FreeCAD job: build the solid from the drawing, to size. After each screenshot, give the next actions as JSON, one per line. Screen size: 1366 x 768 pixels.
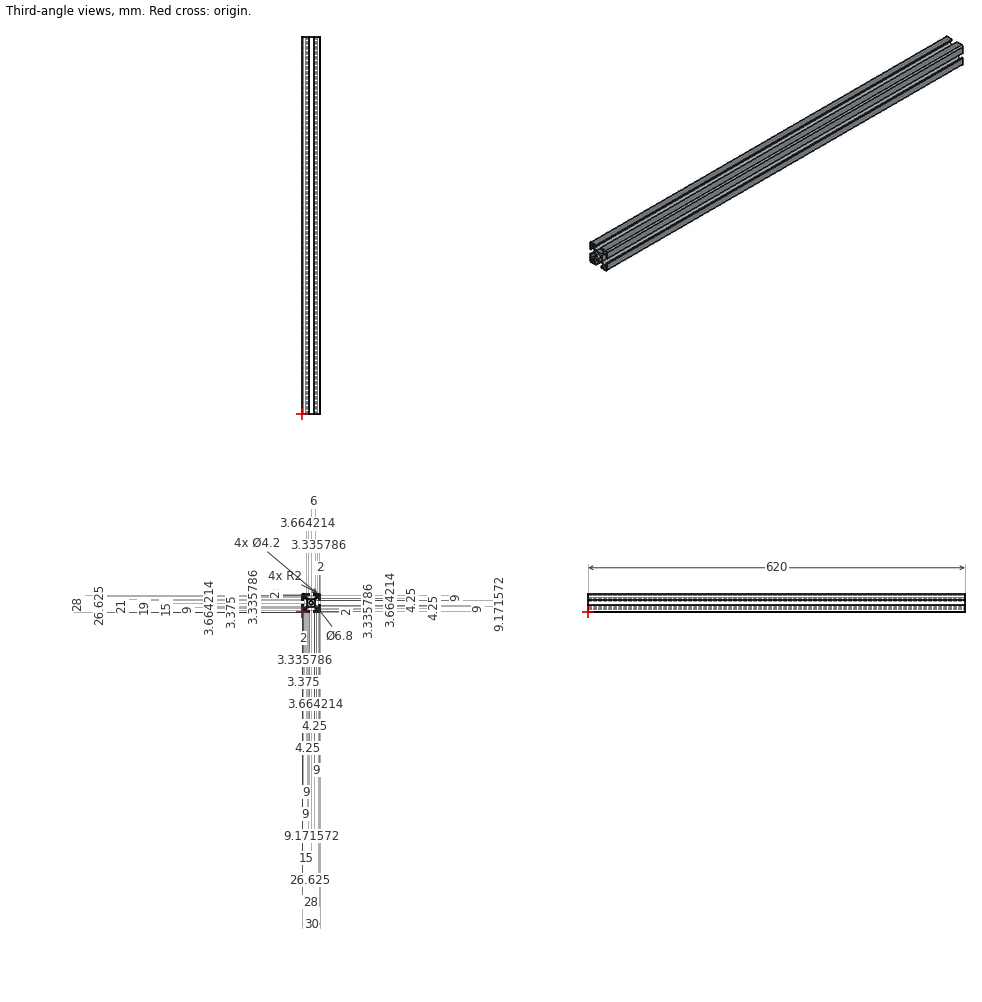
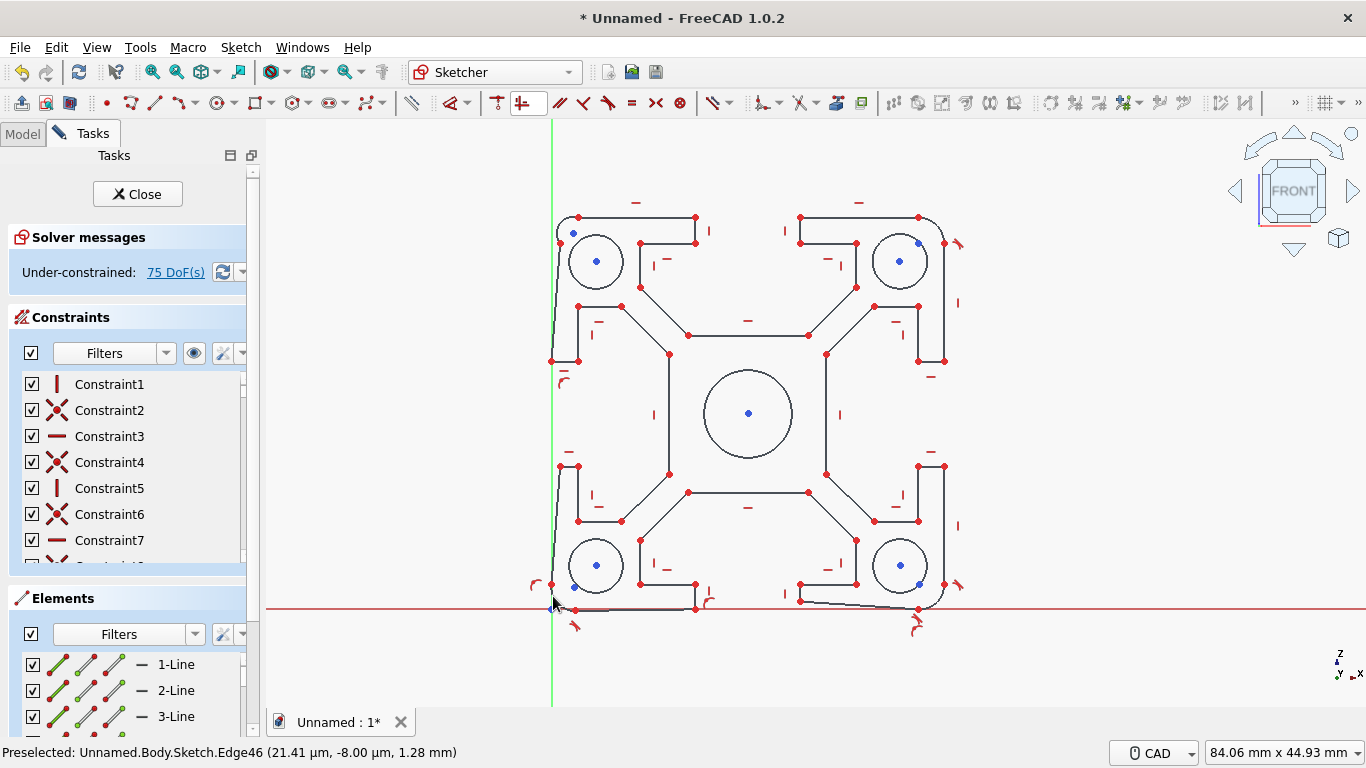
{"action": "left_click", "coordinate": [554, 549]}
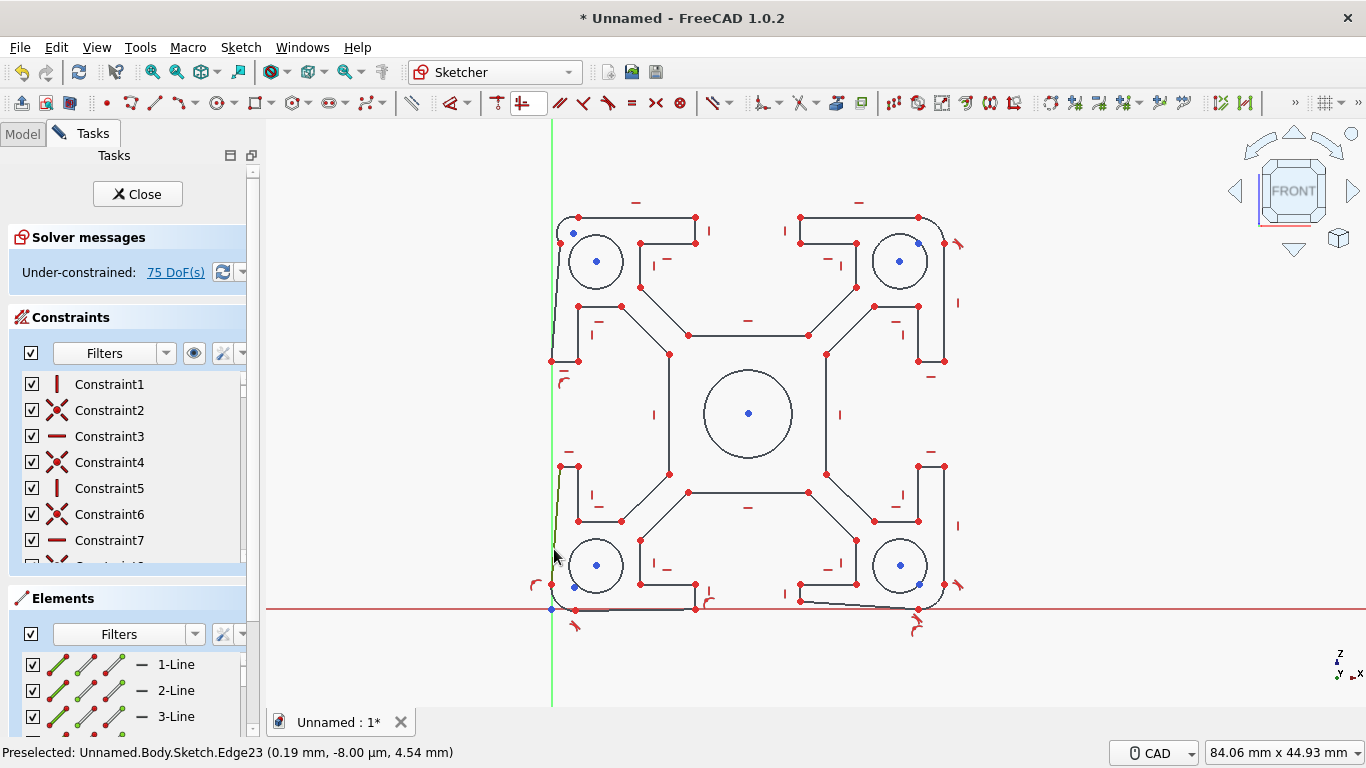
{"action": "left_click", "coordinate": [553, 596]}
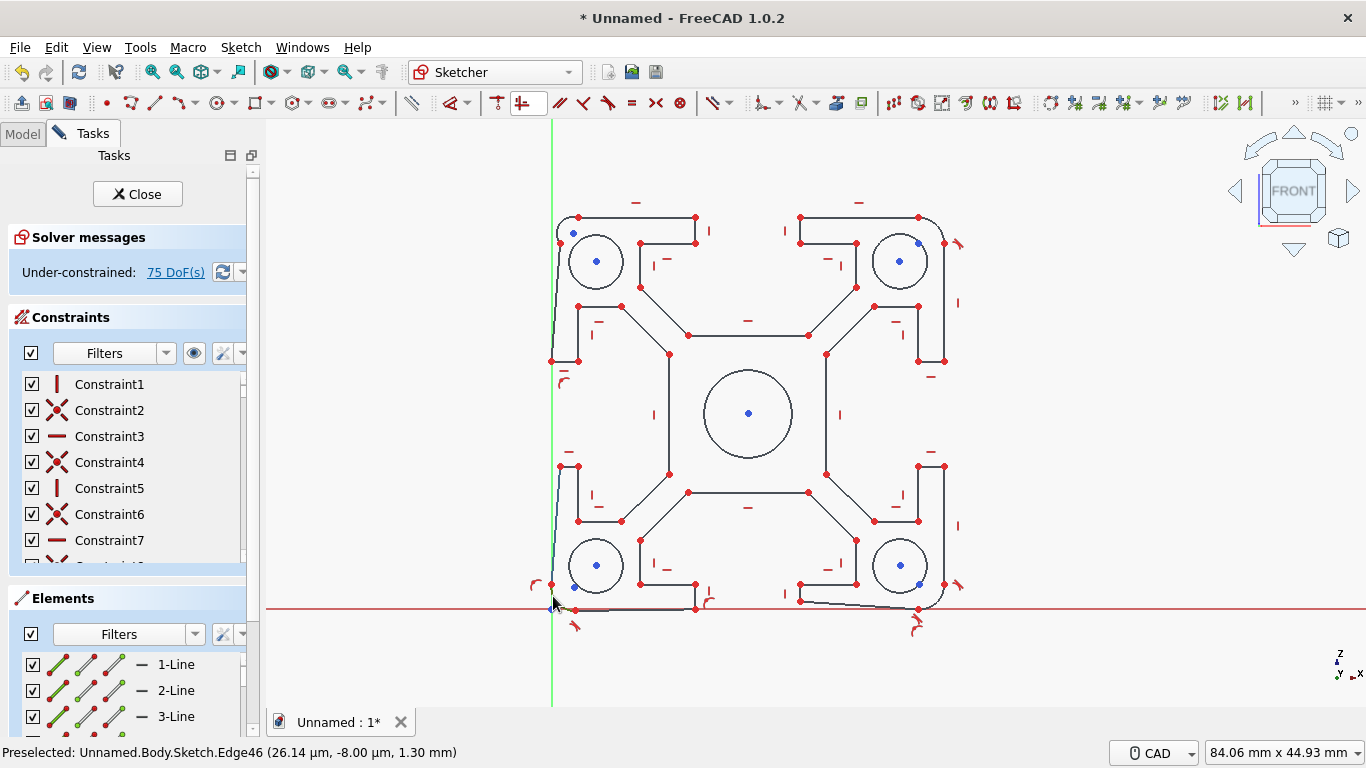
{"action": "key", "text": "t"}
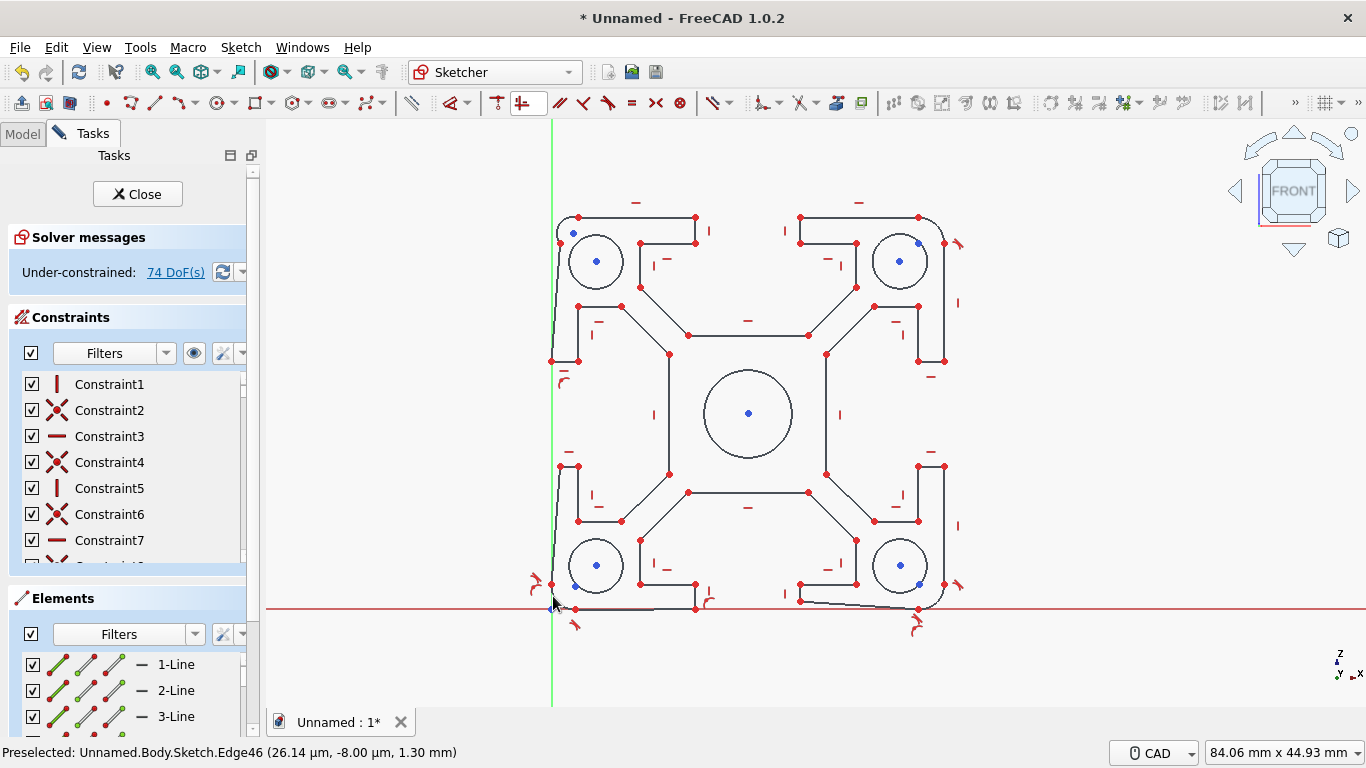
{"action": "left_click", "coordinate": [554, 326]}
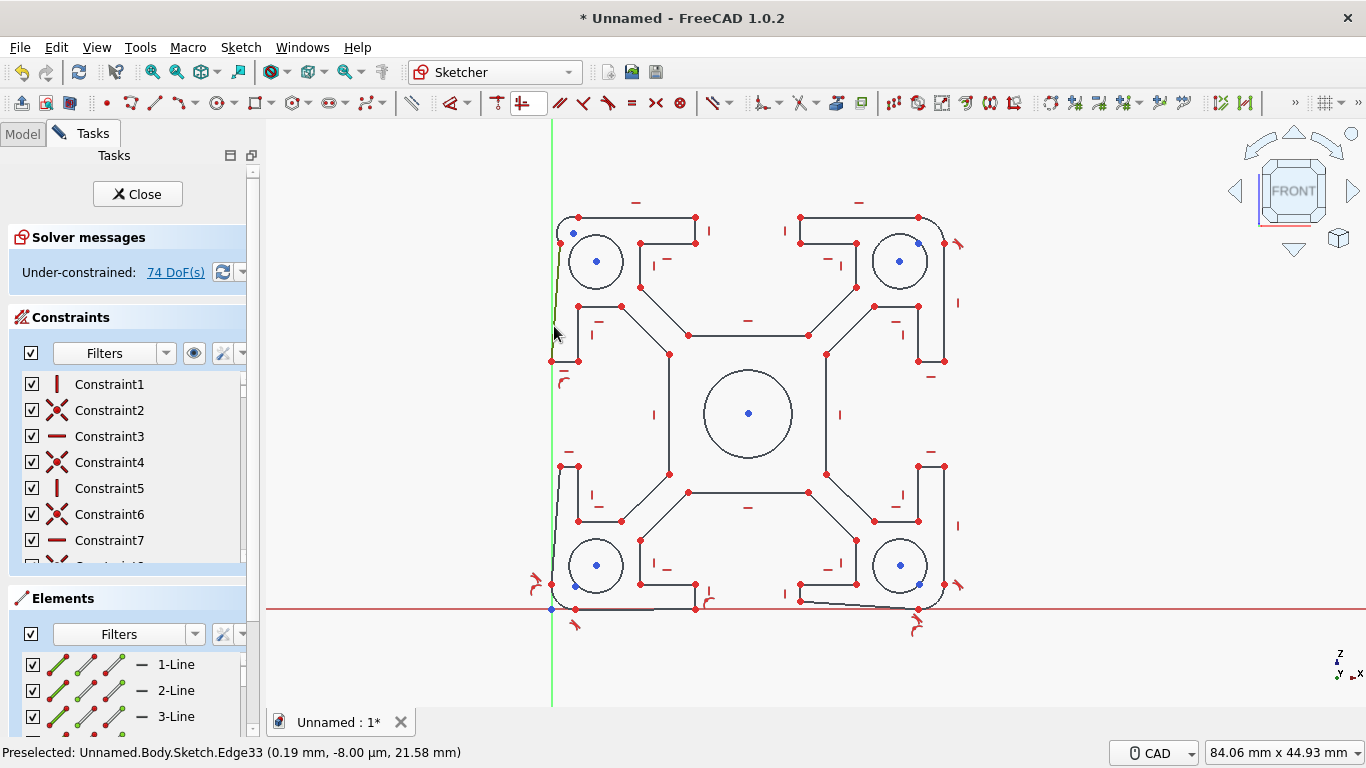
{"action": "left_click", "coordinate": [566, 219]}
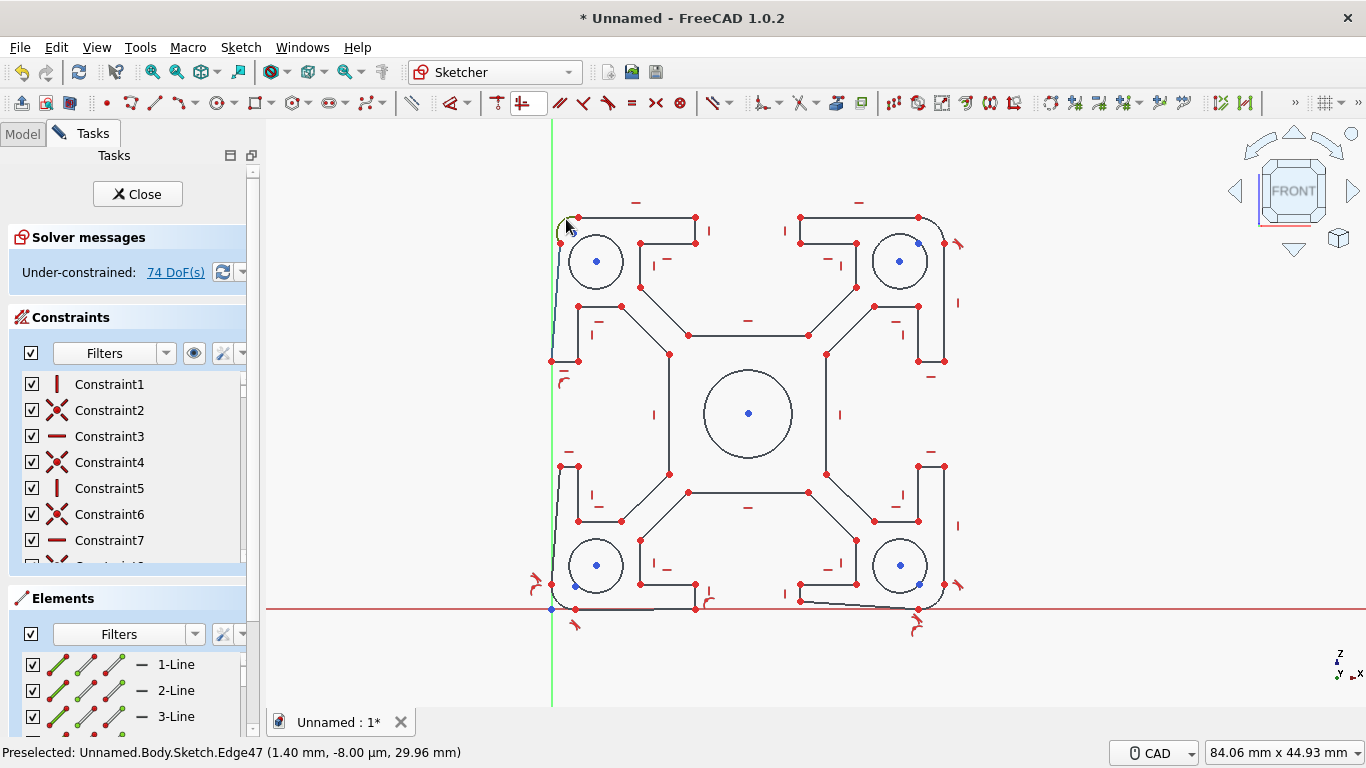
{"action": "key", "text": "t"}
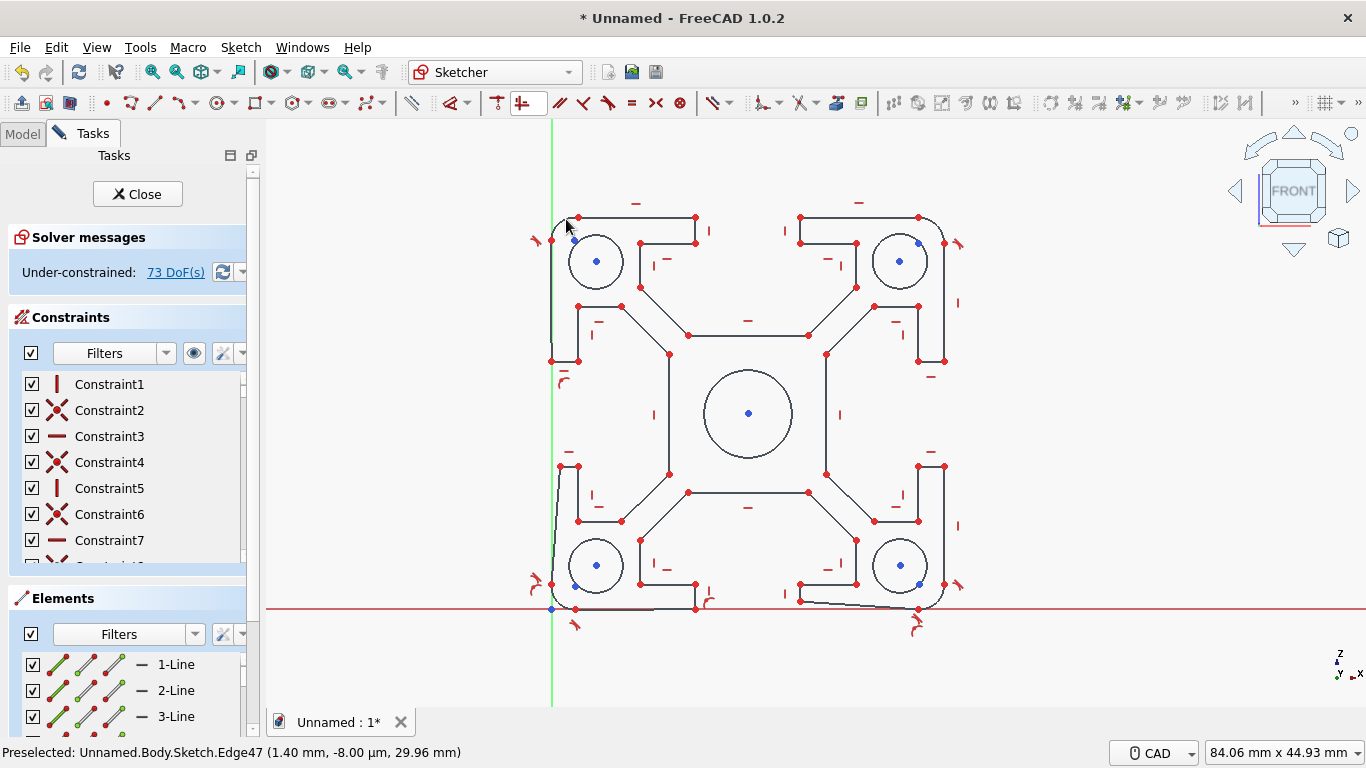
{"action": "left_click", "coordinate": [613, 218]}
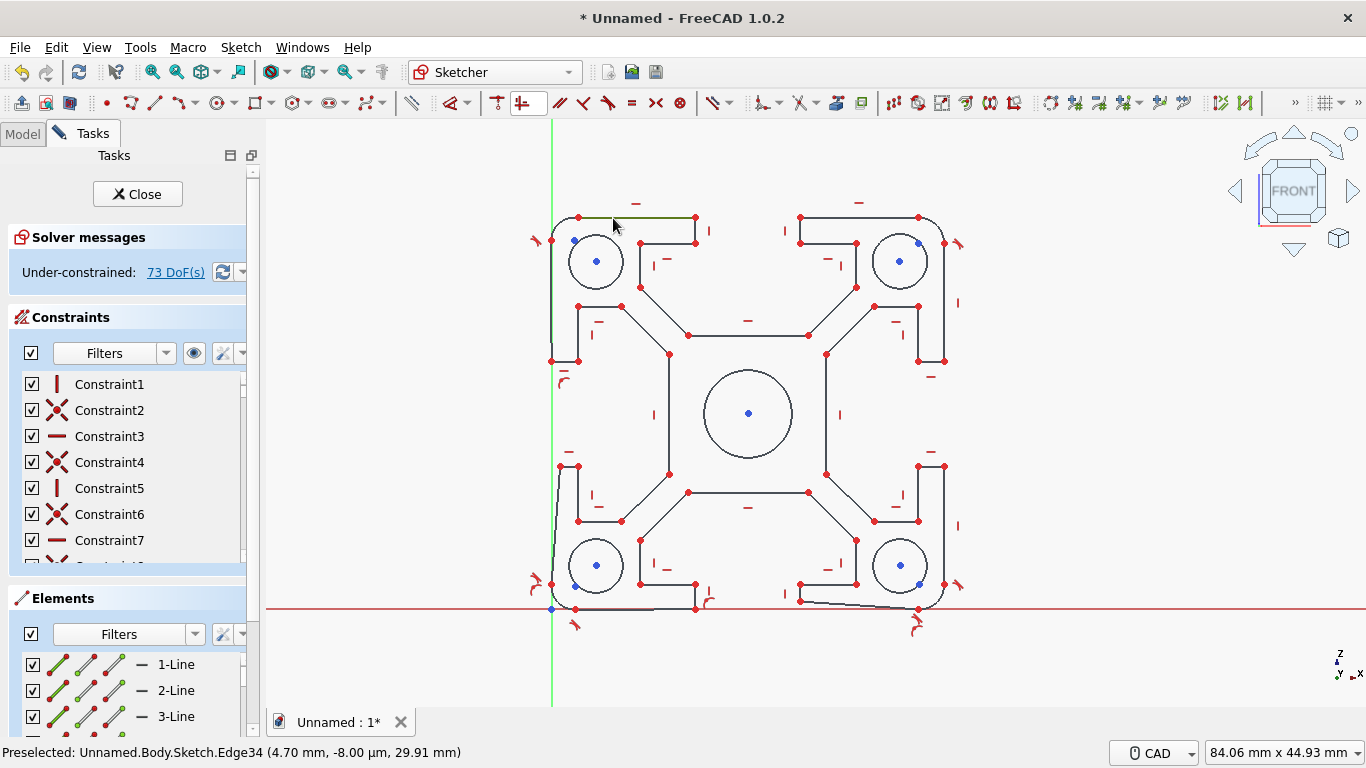
{"action": "left_click", "coordinate": [566, 219]}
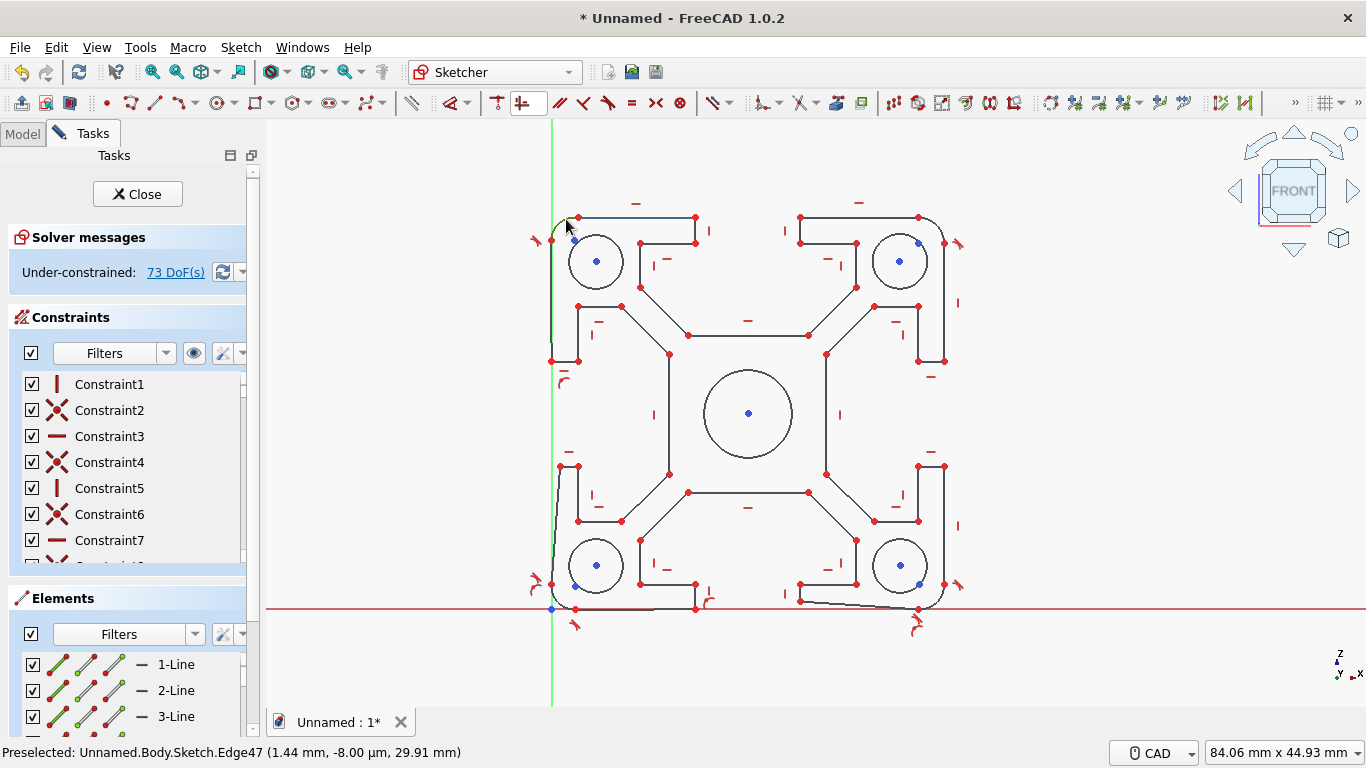
{"action": "key", "text": "t"}